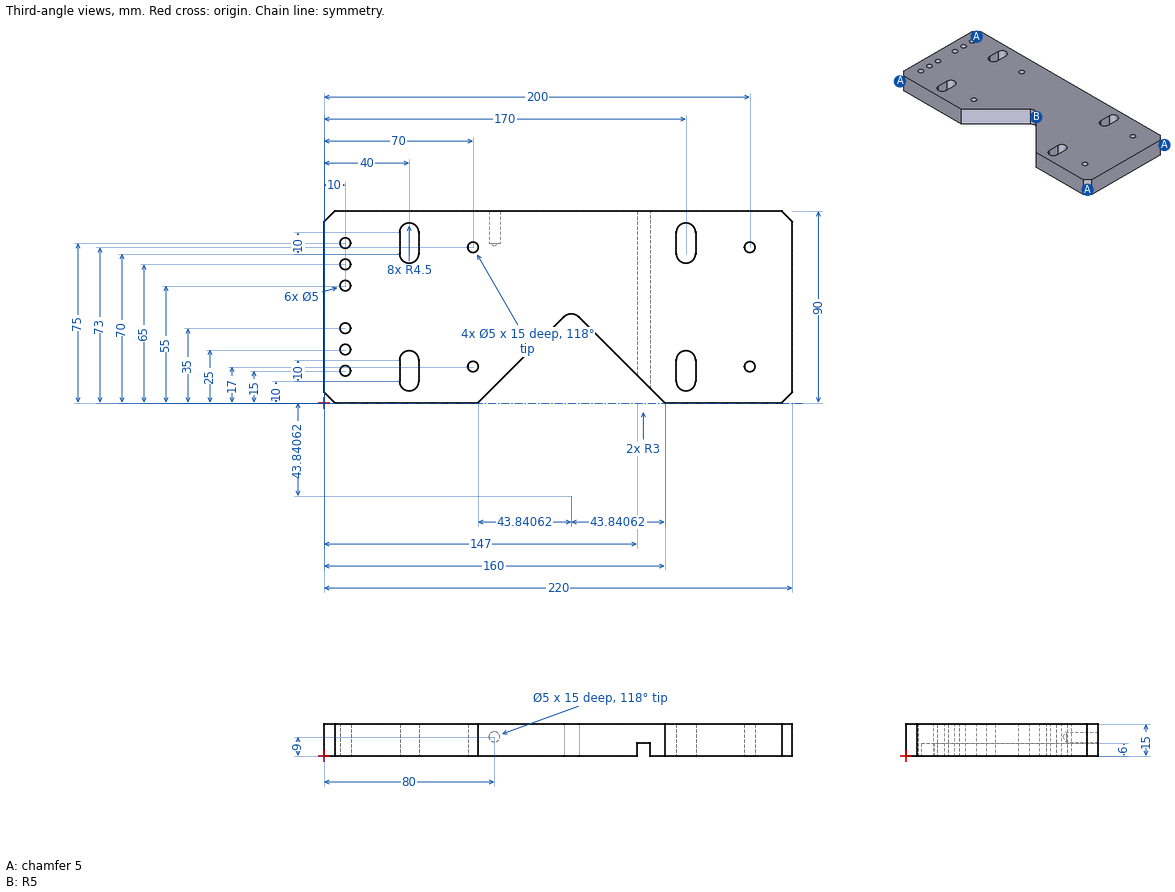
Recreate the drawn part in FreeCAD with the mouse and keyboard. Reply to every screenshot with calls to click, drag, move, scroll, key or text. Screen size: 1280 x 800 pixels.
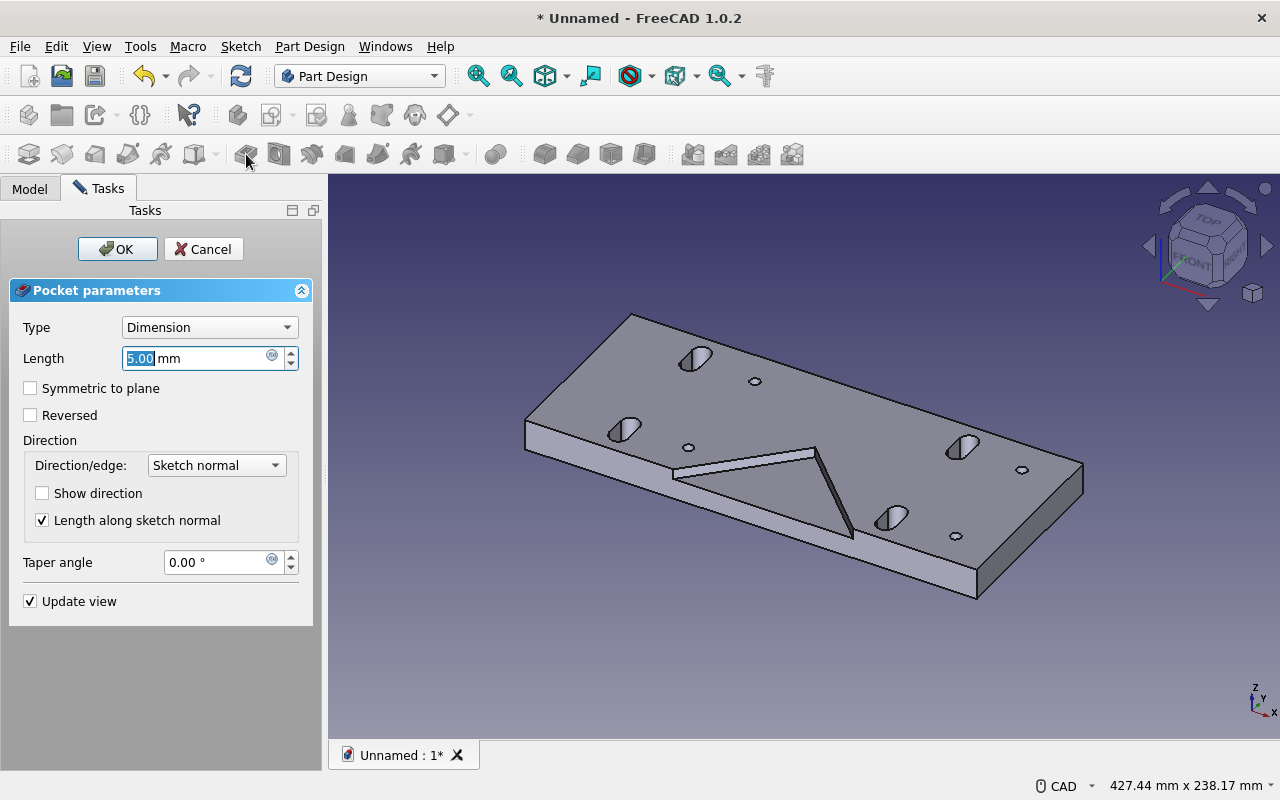
click(210, 328)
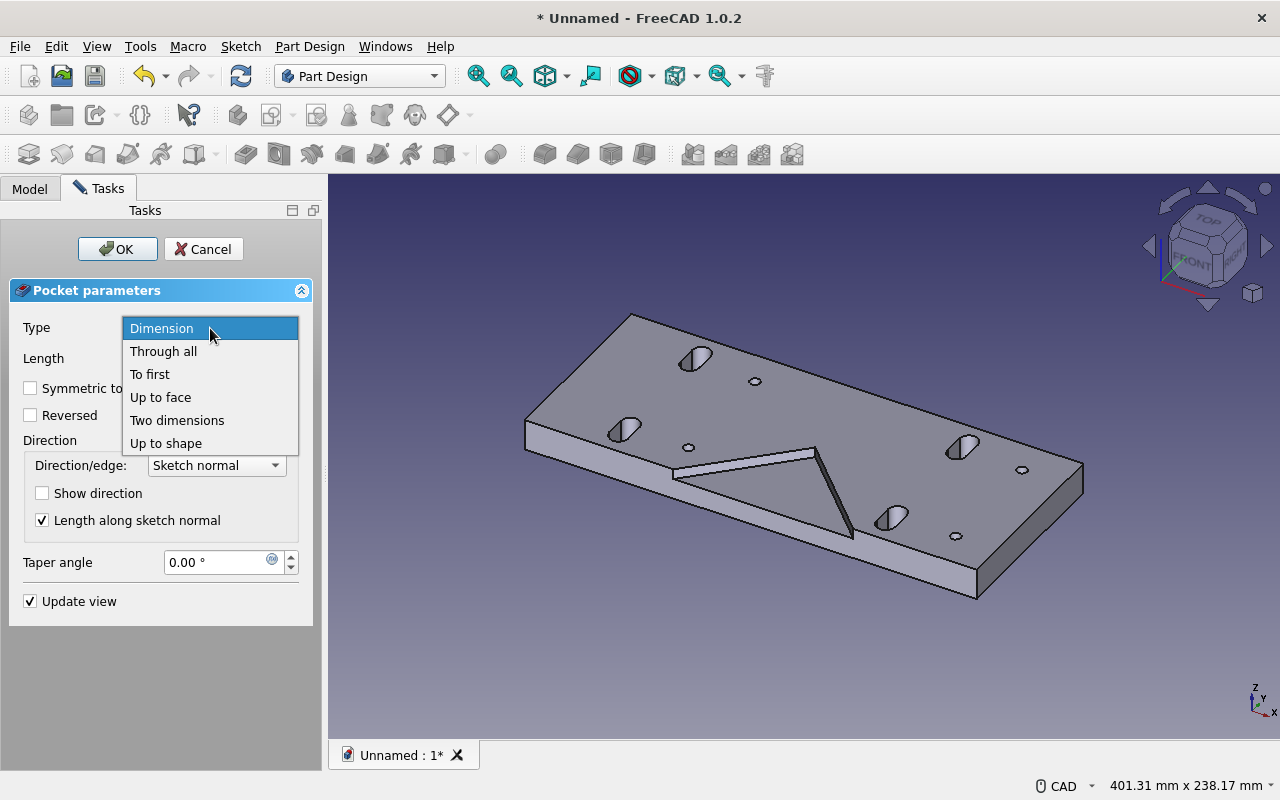
click(208, 352)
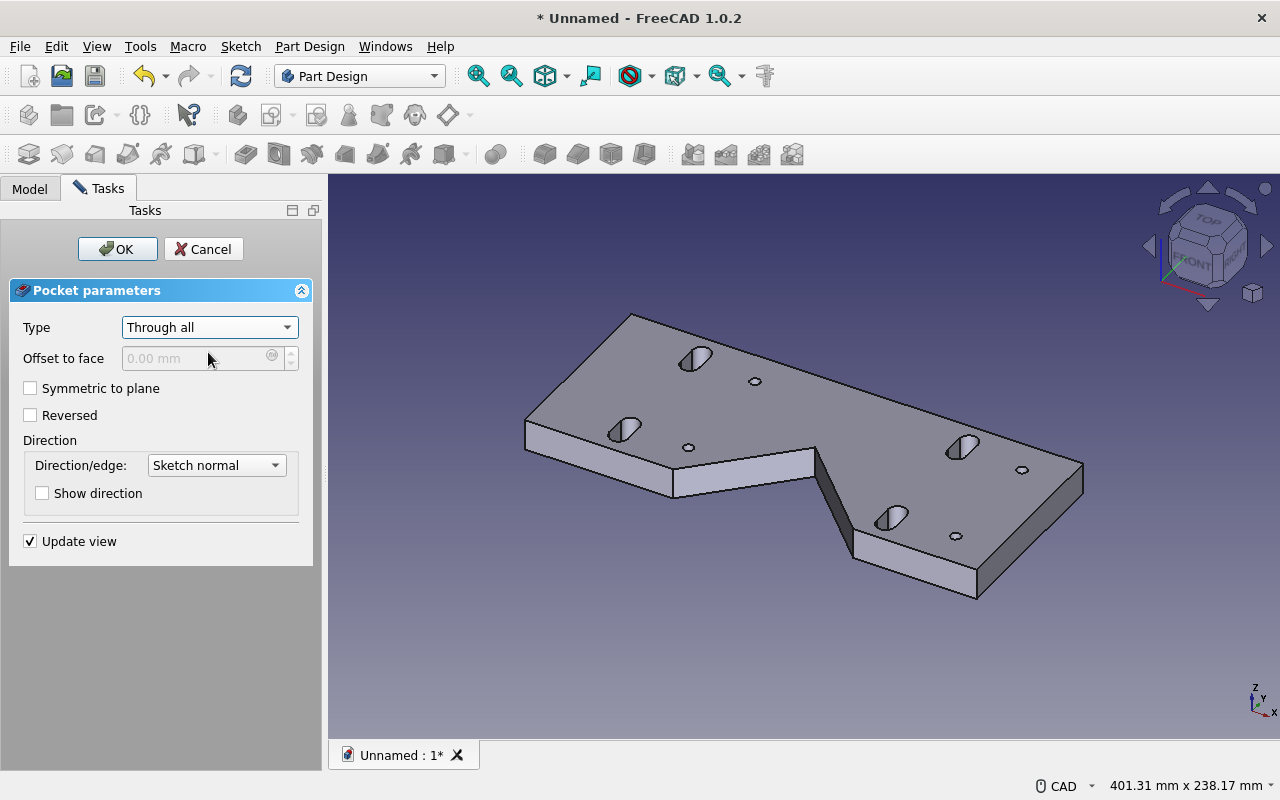
click(118, 249)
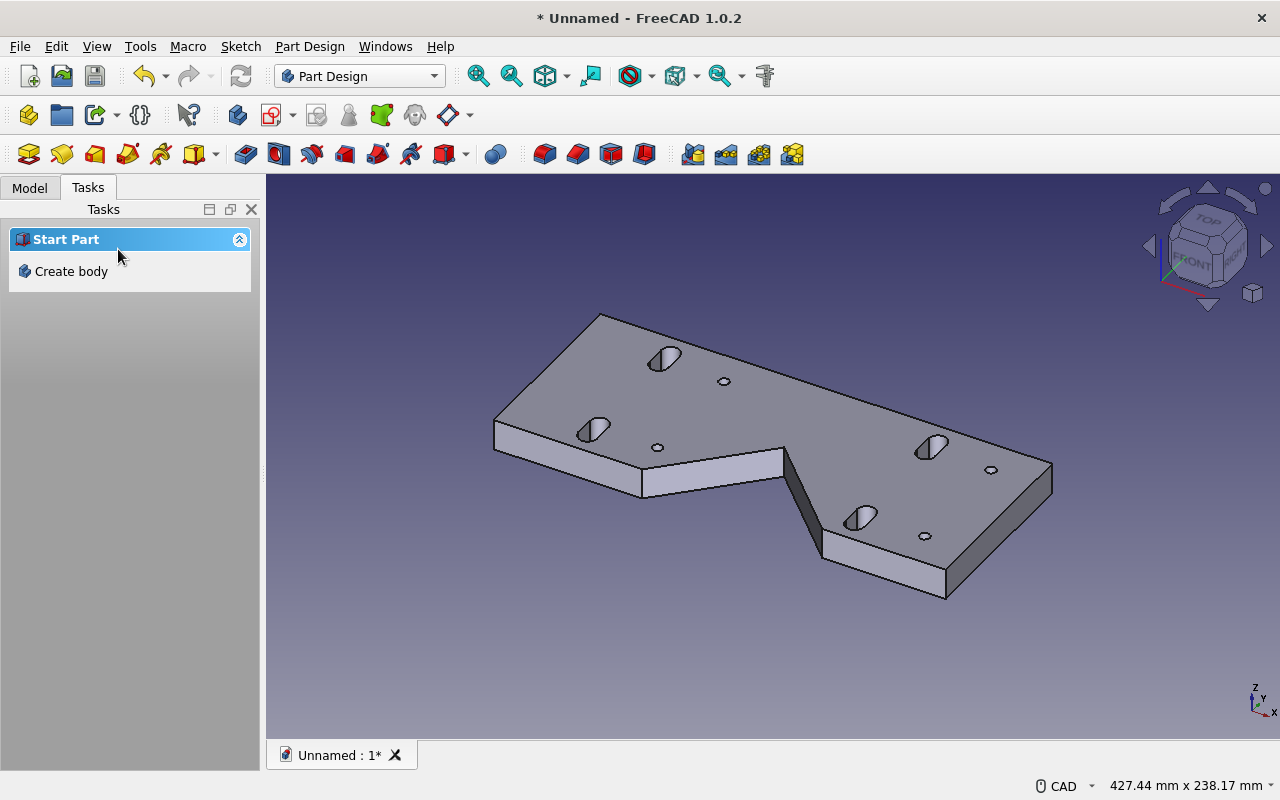
key(4)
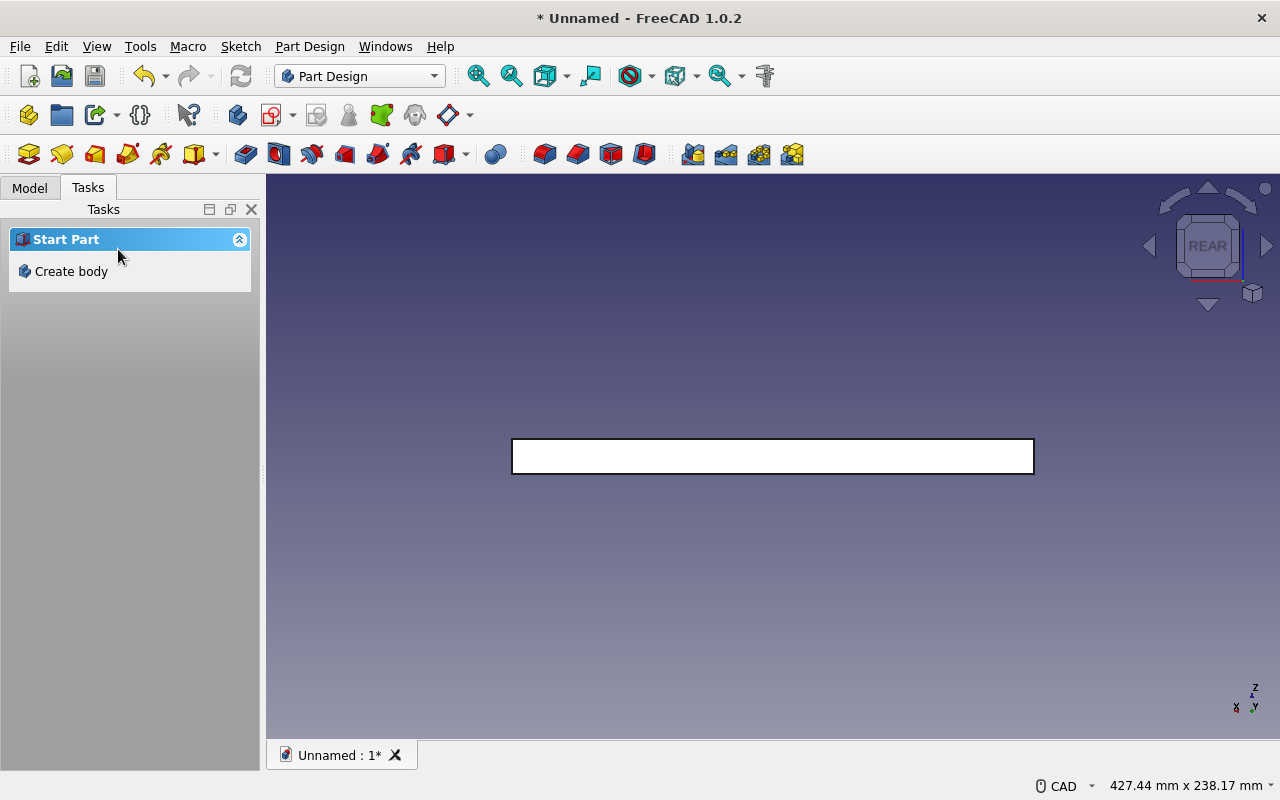
click(549, 455)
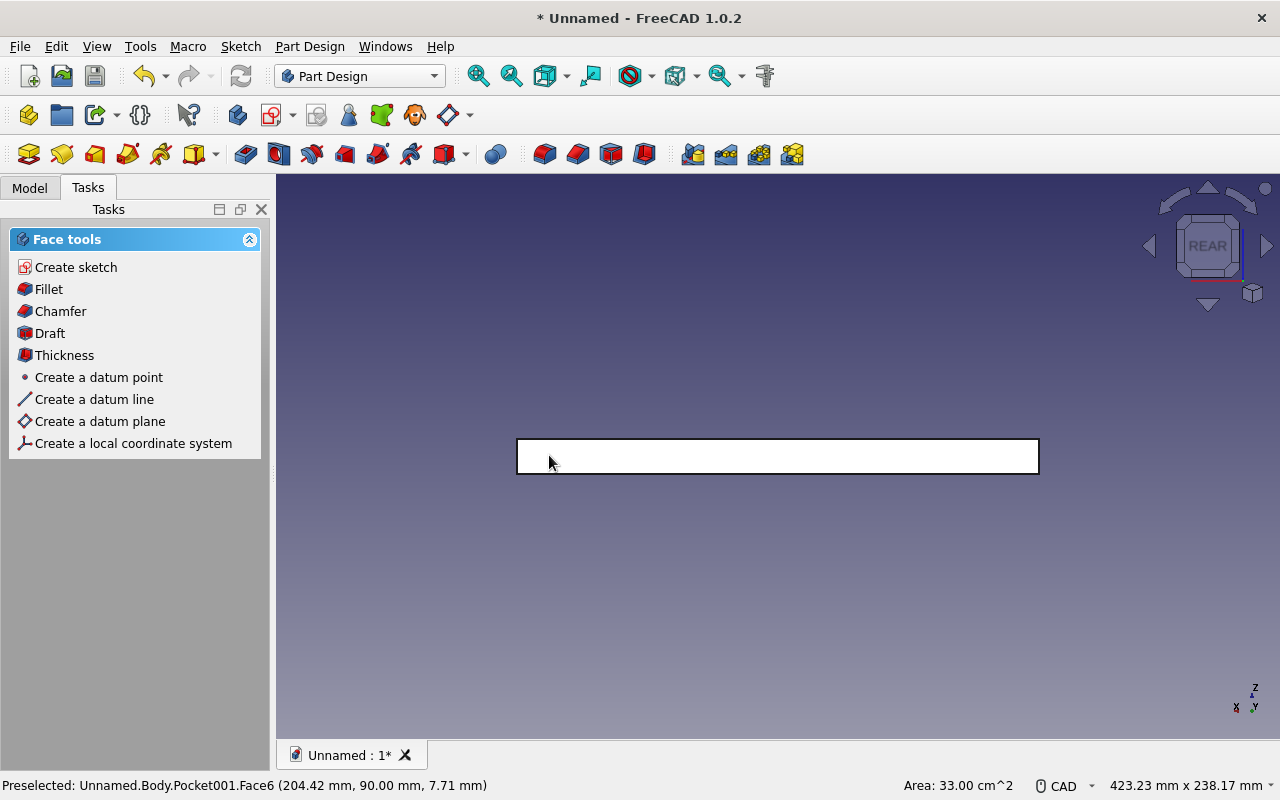
click(270, 116)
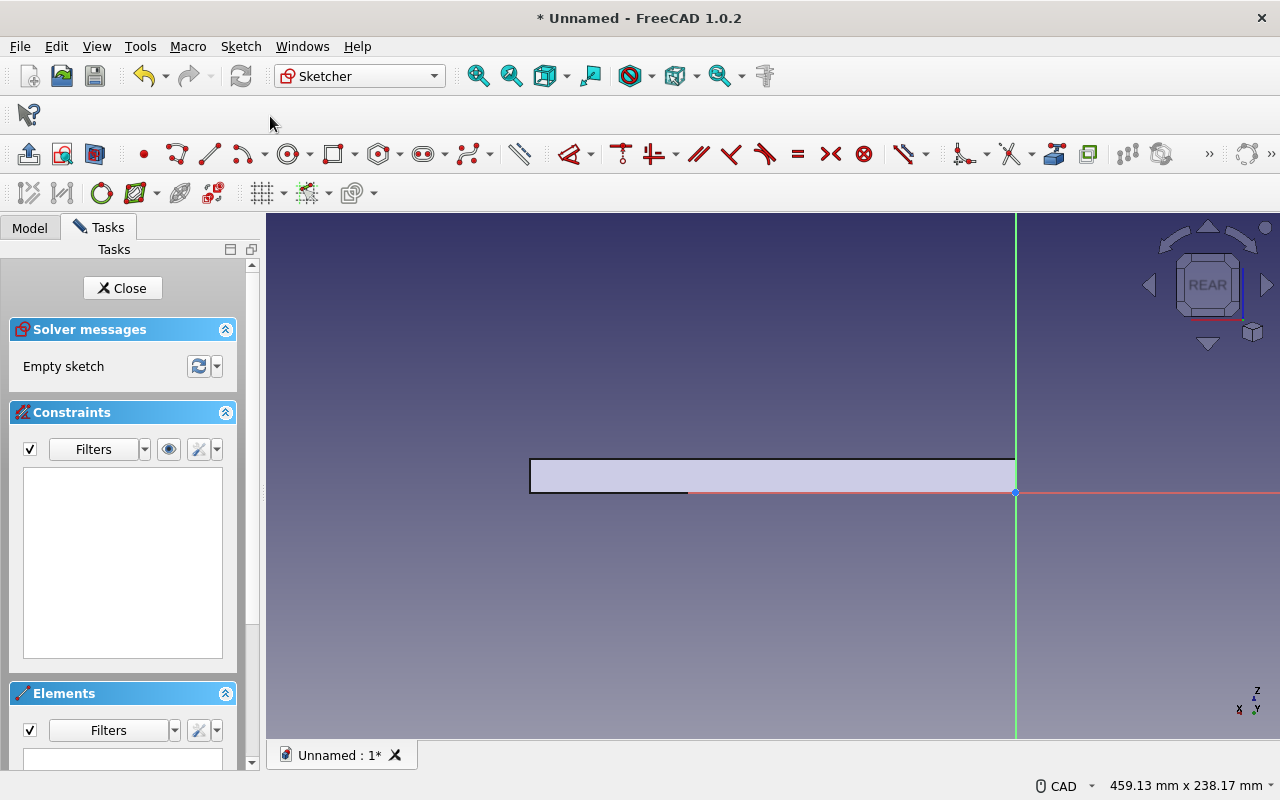
scroll(846, 473, up, 15)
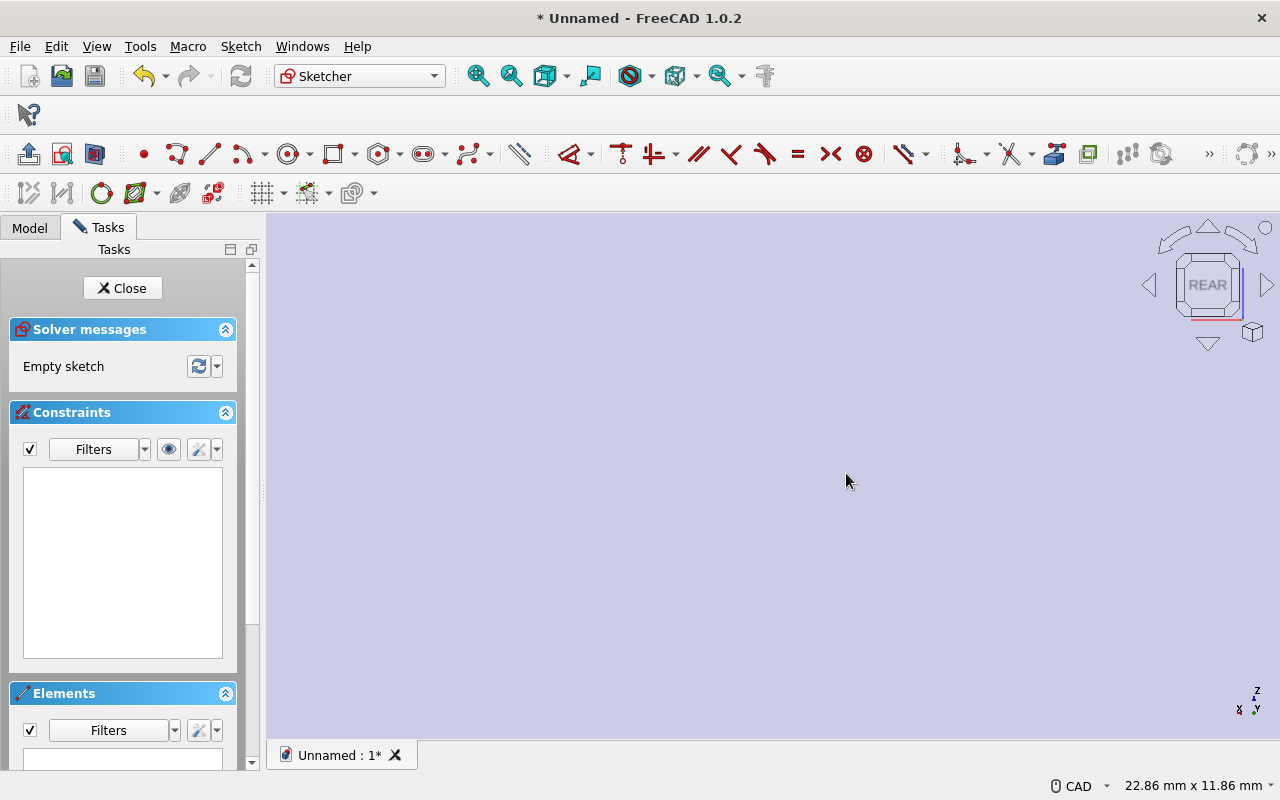
scroll(690, 419, up, 2)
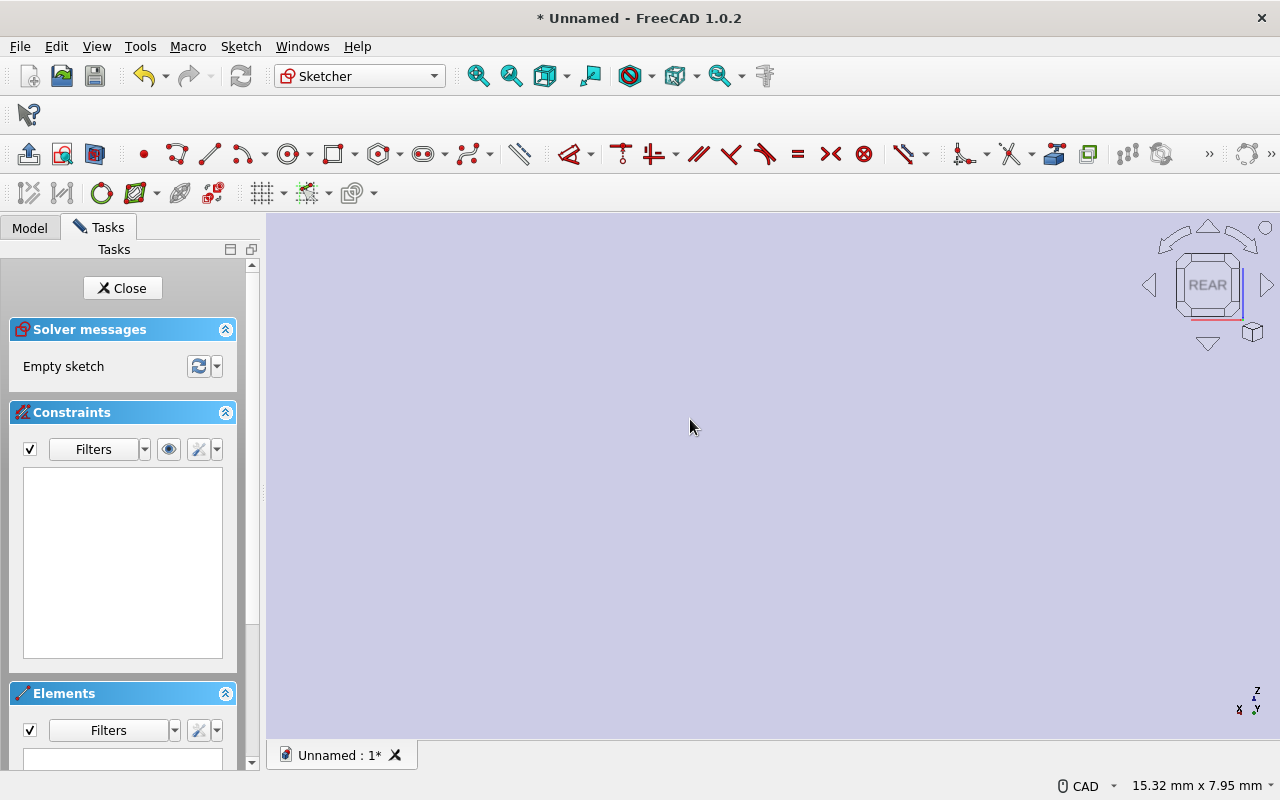
key(g)
key(c)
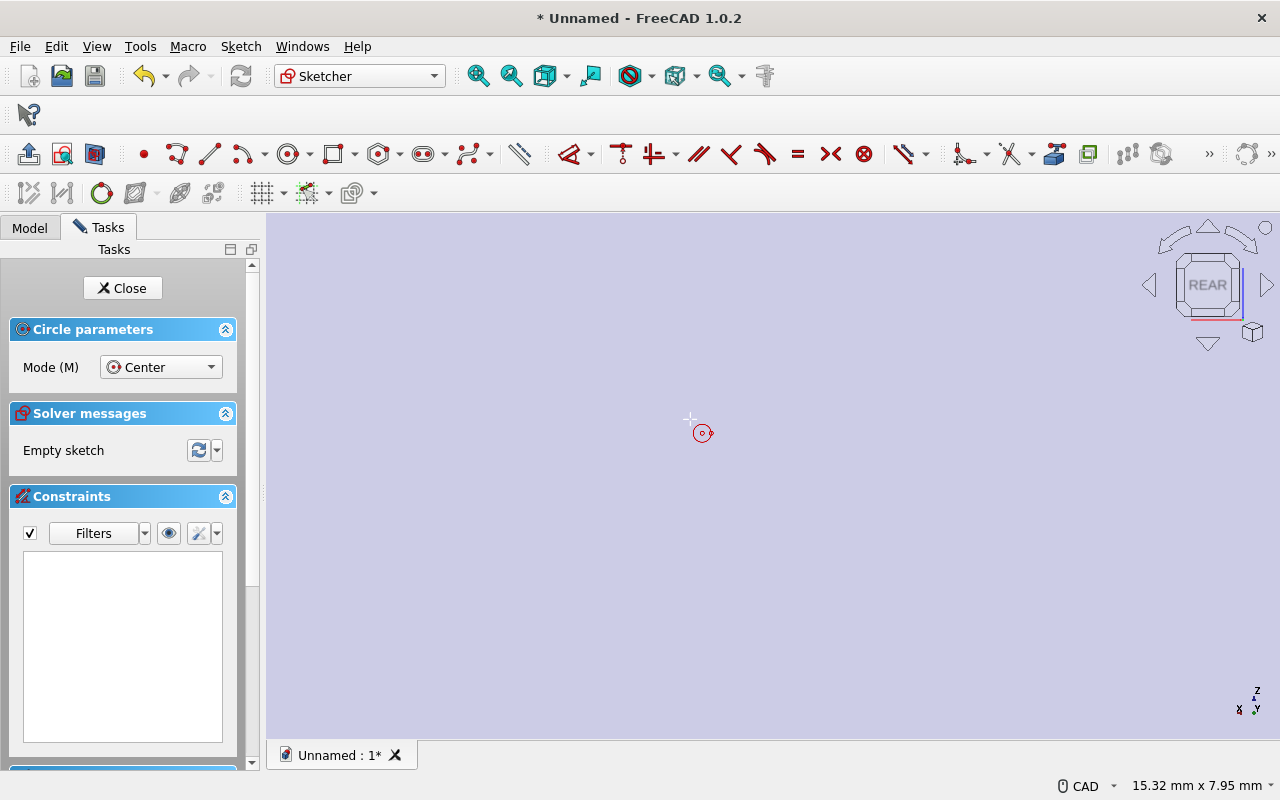
click(704, 476)
click(821, 359)
key(Escape)